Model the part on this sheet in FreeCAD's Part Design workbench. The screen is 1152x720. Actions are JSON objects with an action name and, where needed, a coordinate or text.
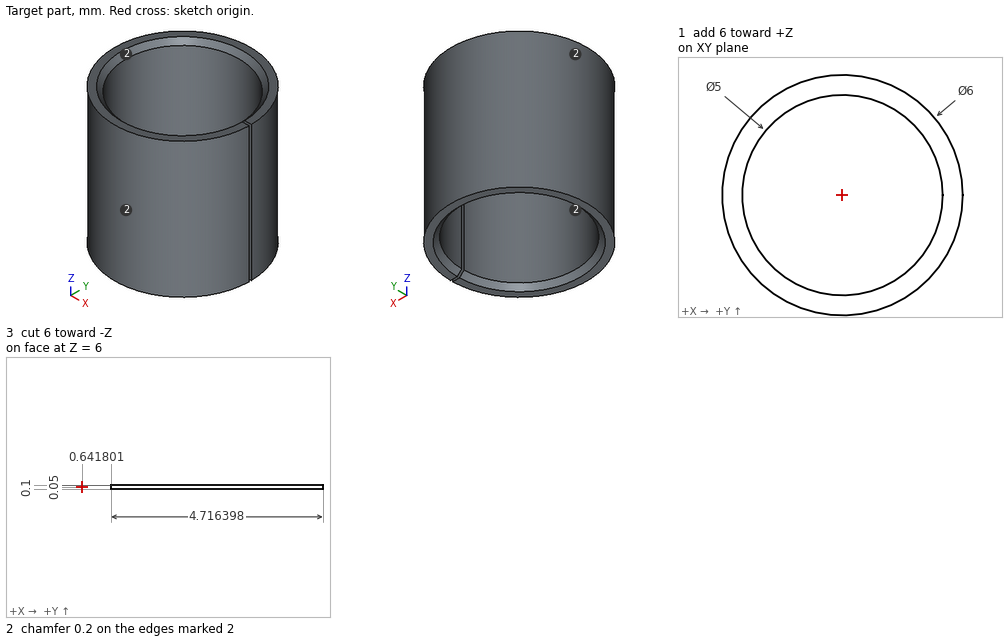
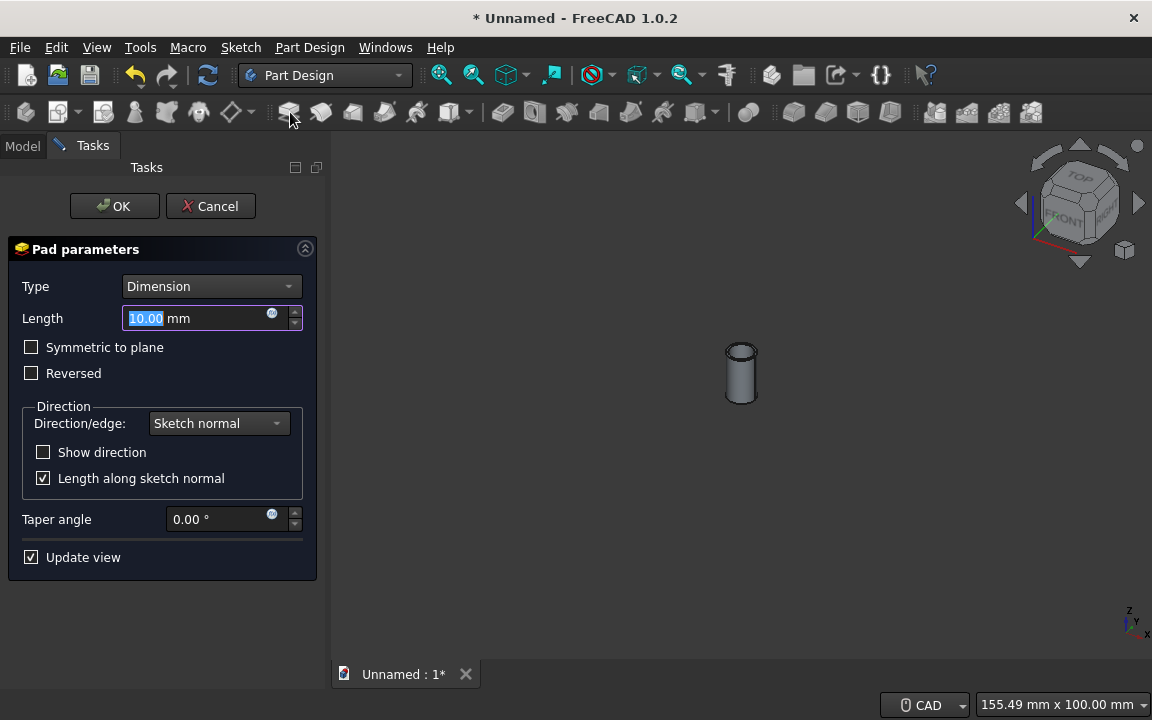
{"action": "type", "text": "6"}
{"action": "key", "text": "Tab"}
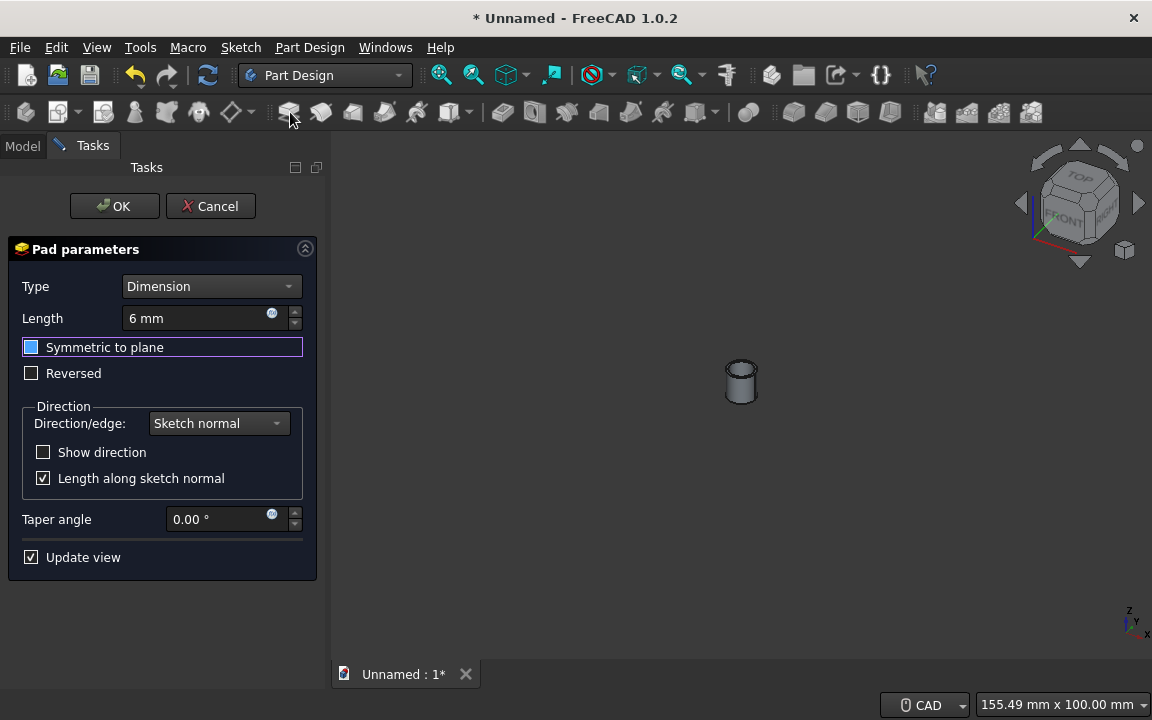
{"action": "left_click", "coordinate": [115, 206]}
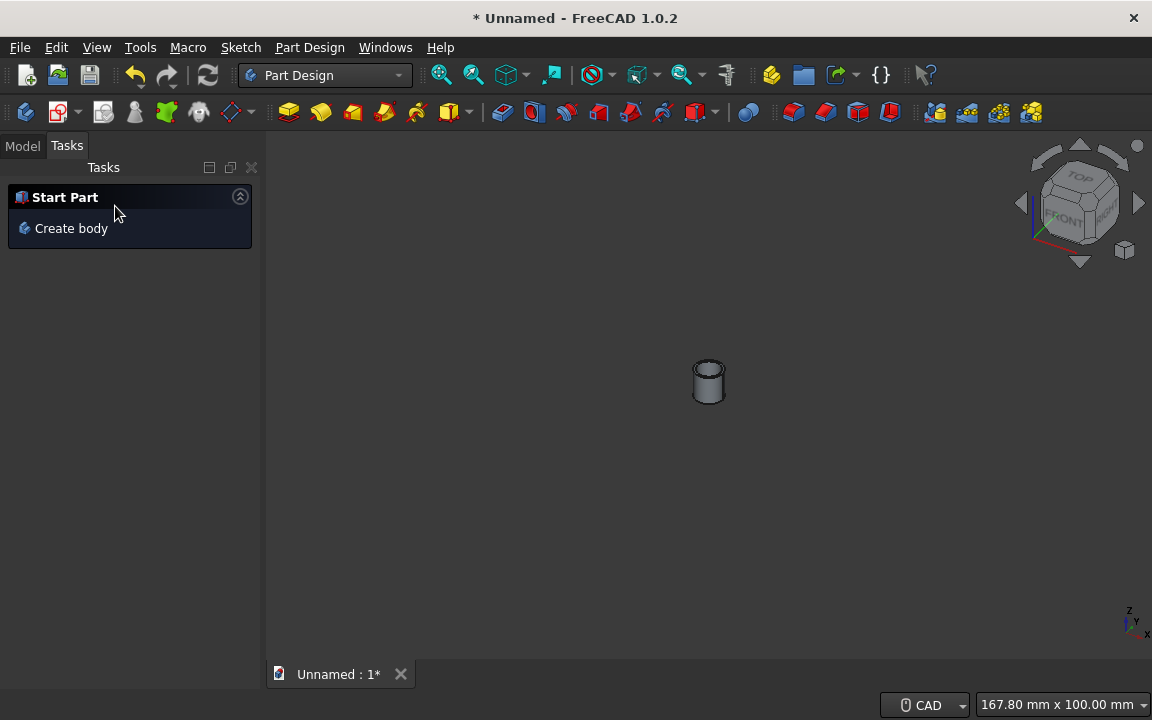
{"action": "left_click", "coordinate": [442, 76]}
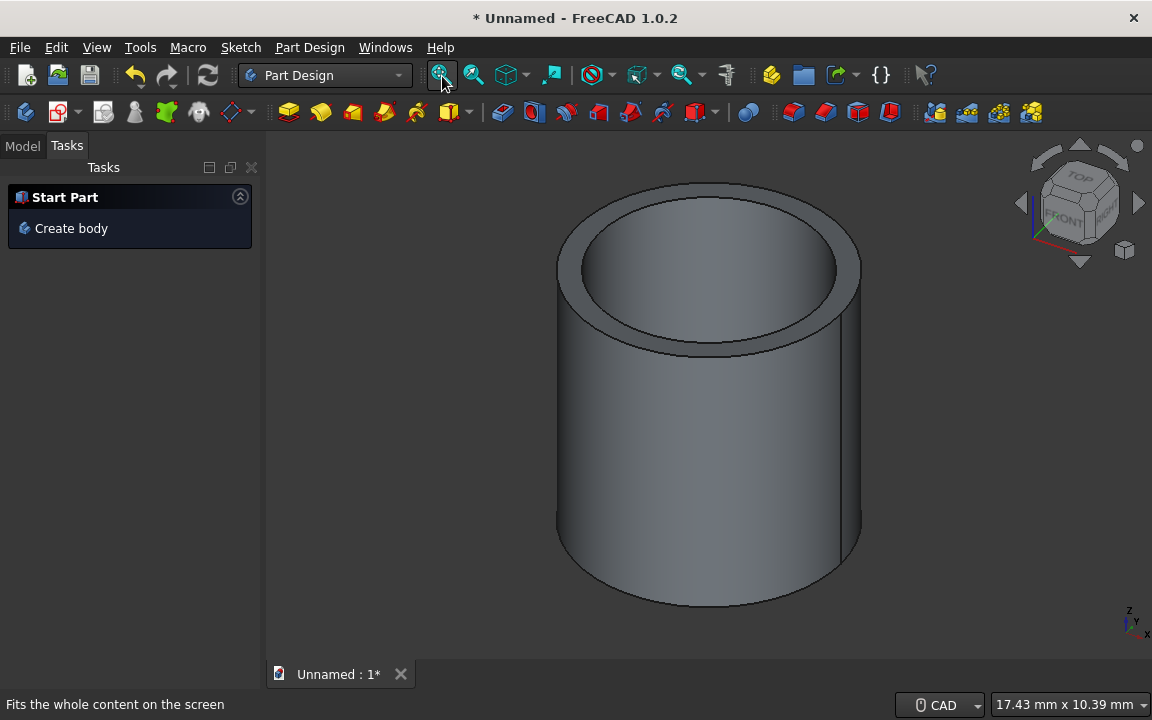
{"action": "left_click", "coordinate": [599, 233]}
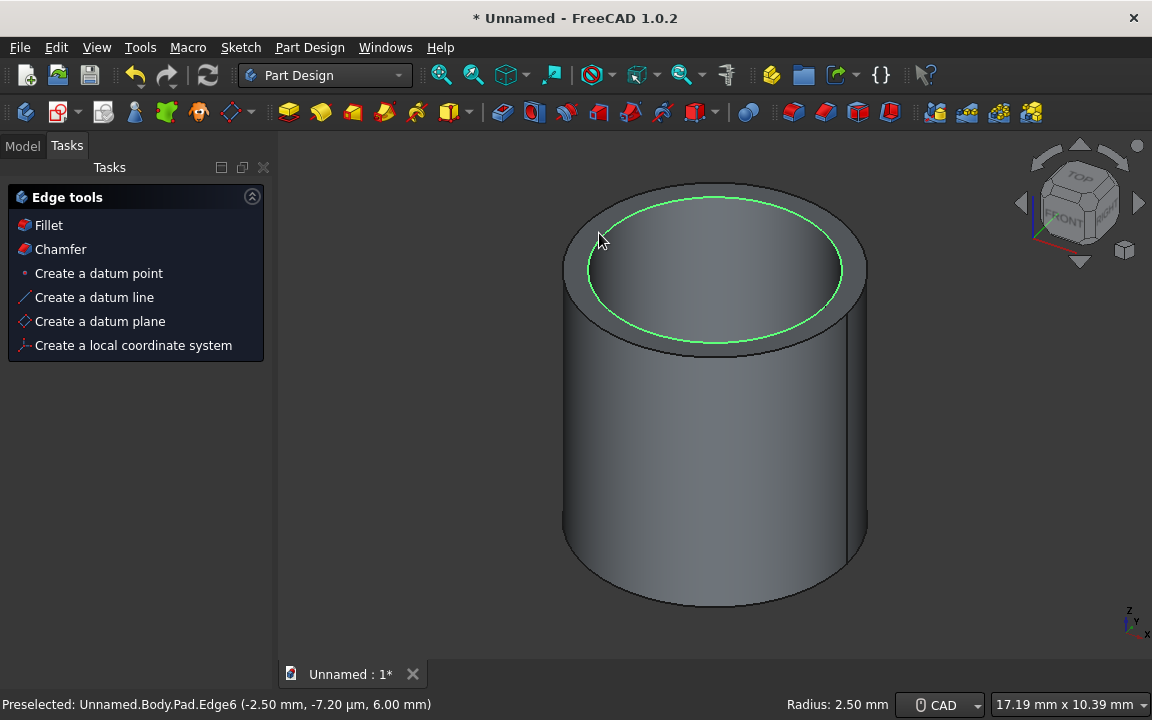
{"action": "key", "text": "0"}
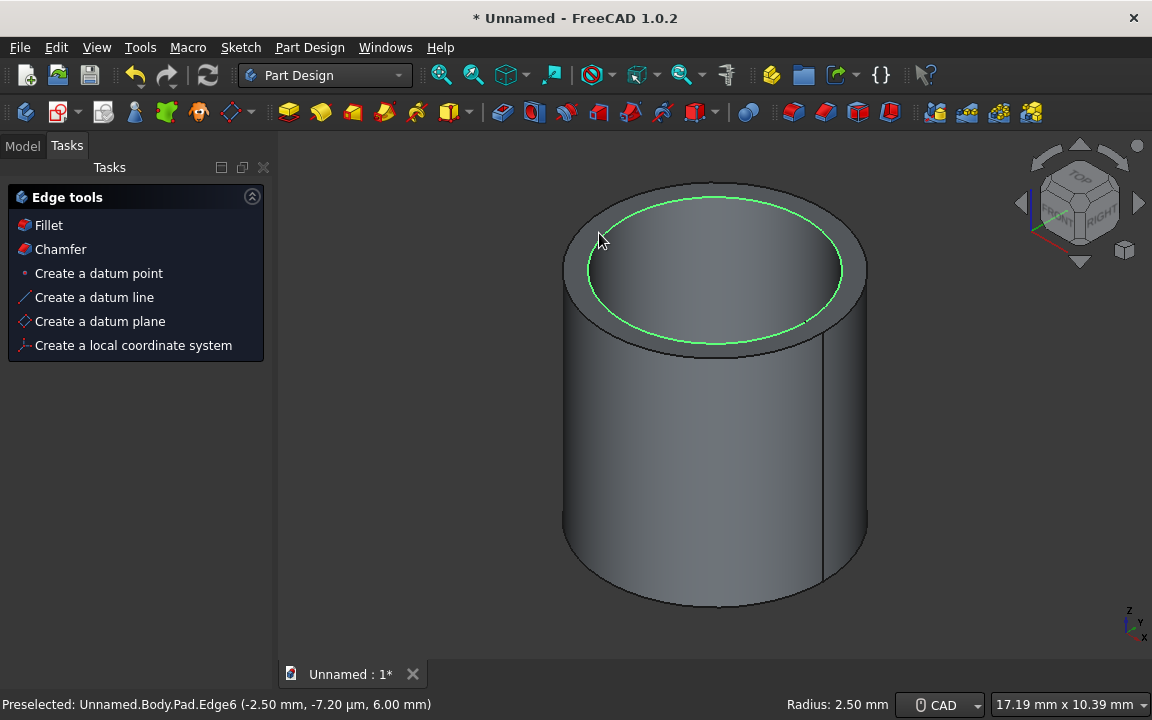
{"action": "key", "text": "2"}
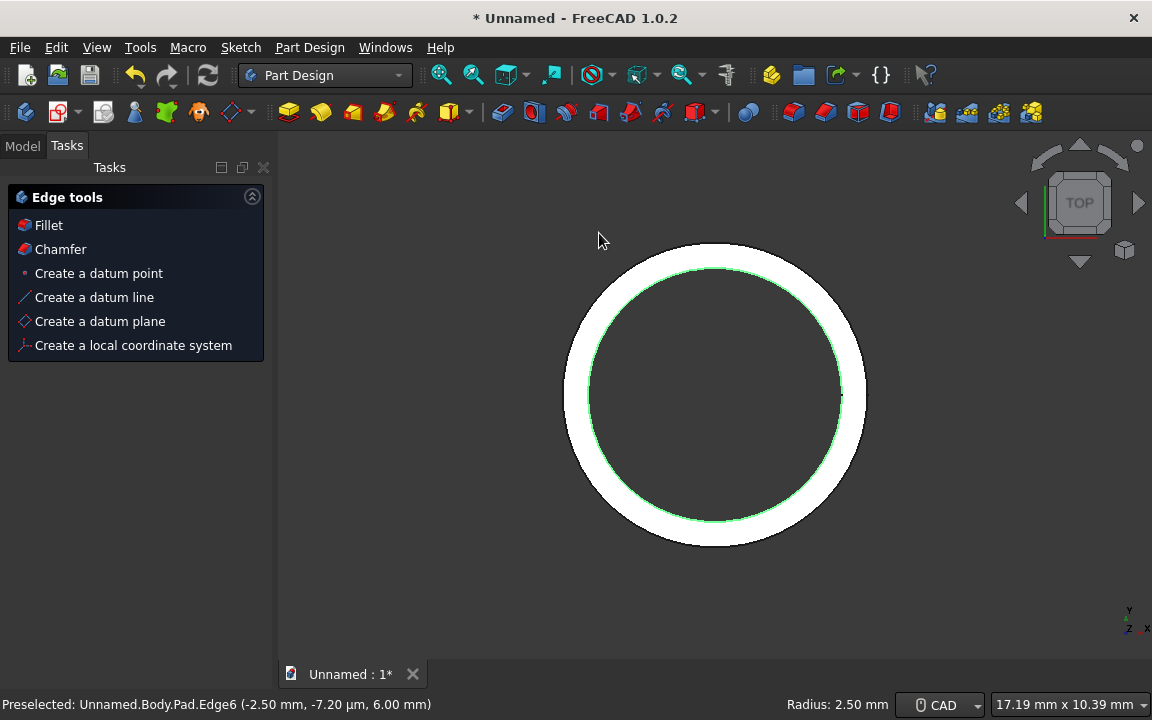
{"action": "key", "text": "1"}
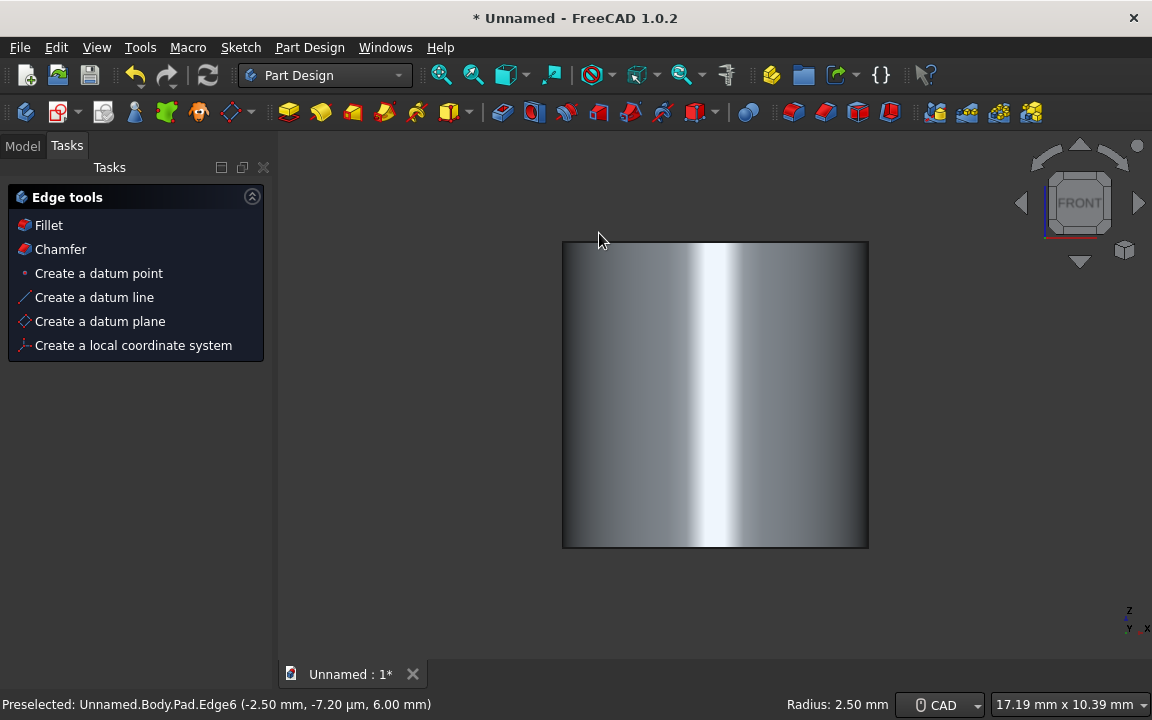
{"action": "key", "text": "3"}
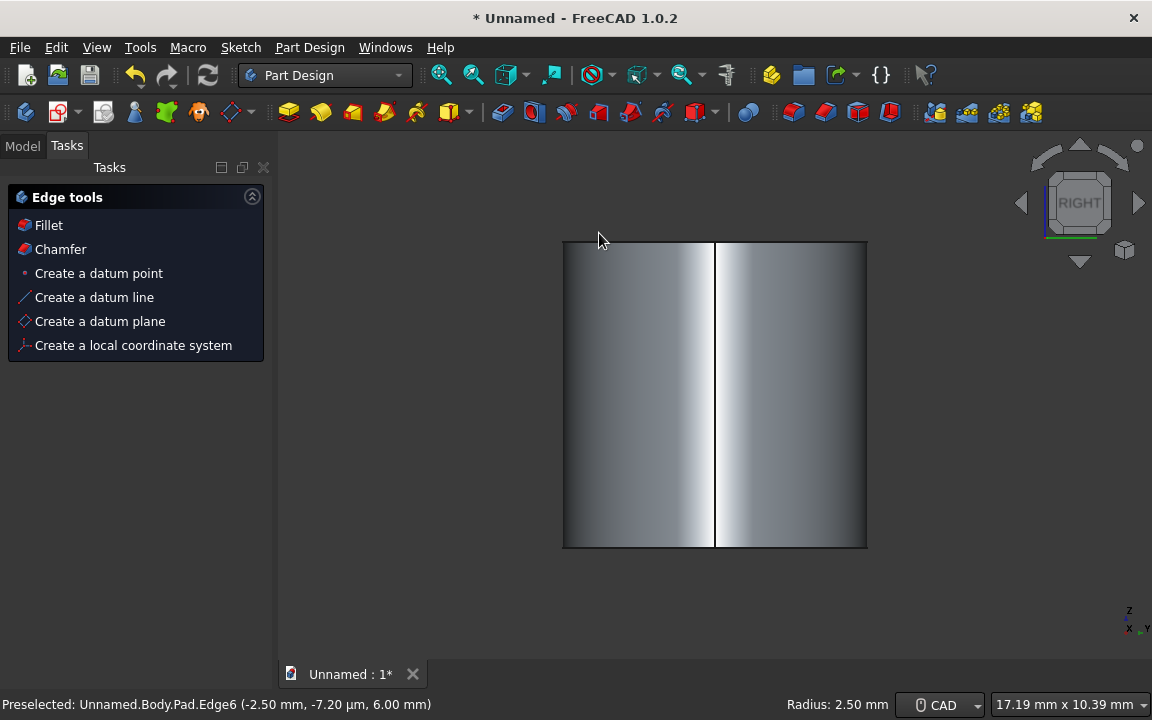
{"action": "key", "text": "5"}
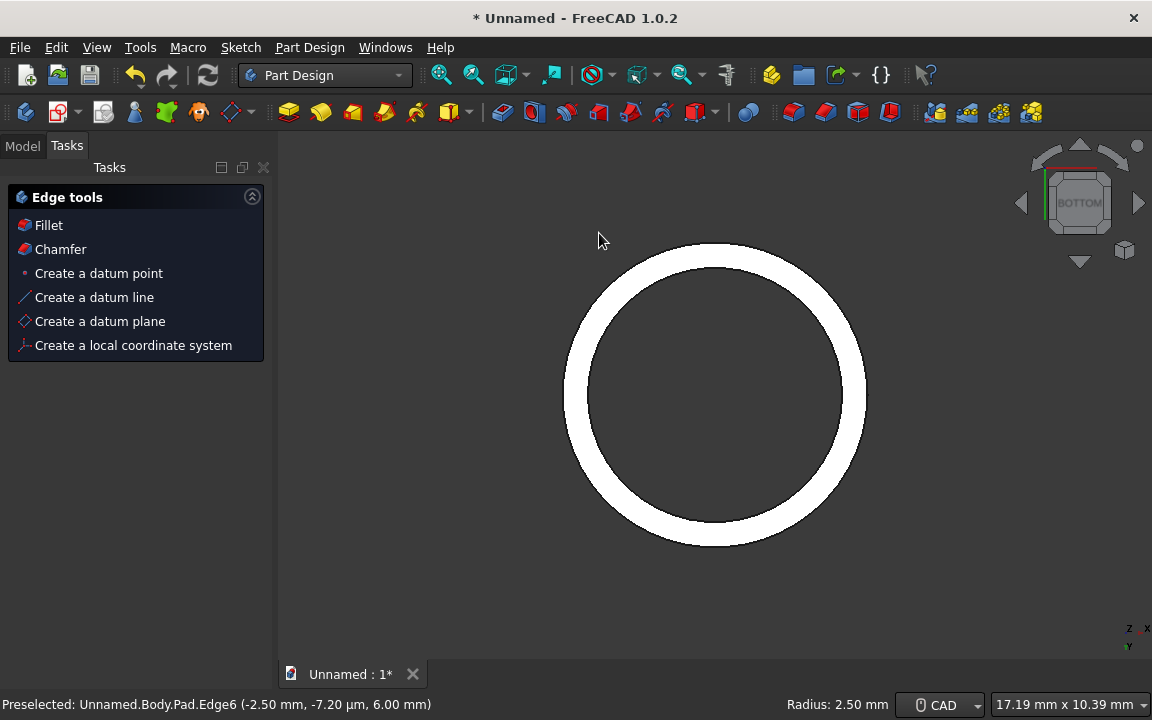
{"action": "left_click", "coordinate": [588, 394], "text": "ctrl"}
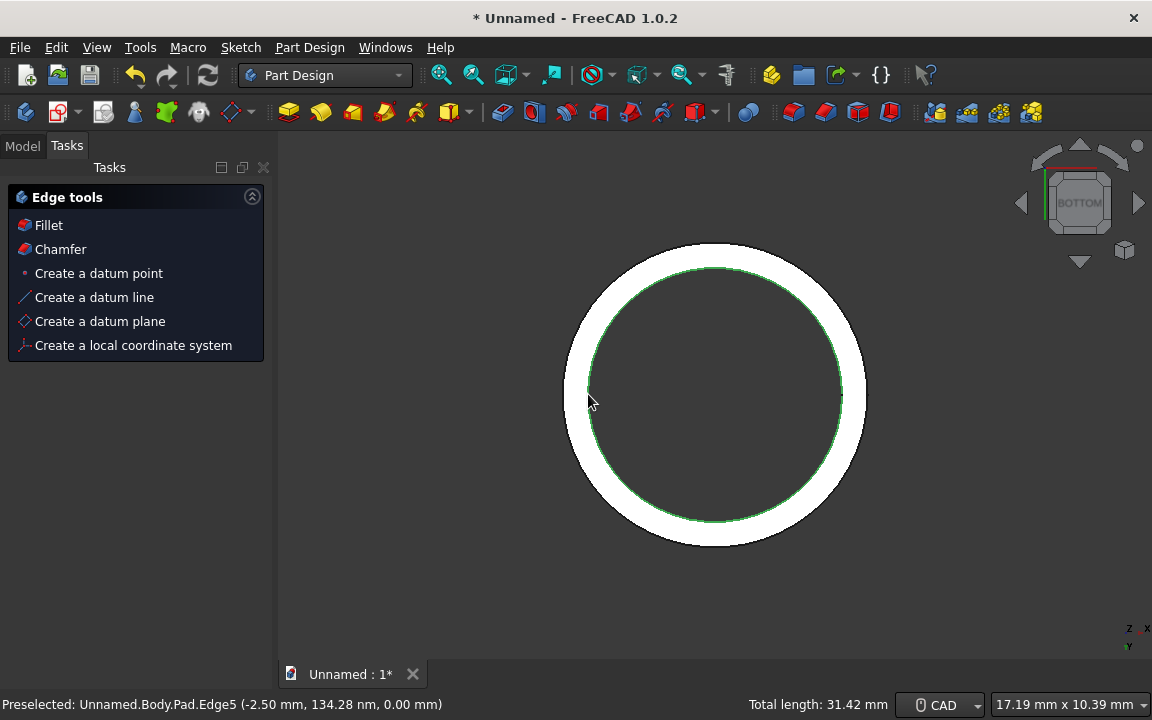
{"action": "left_click", "coordinate": [826, 112]}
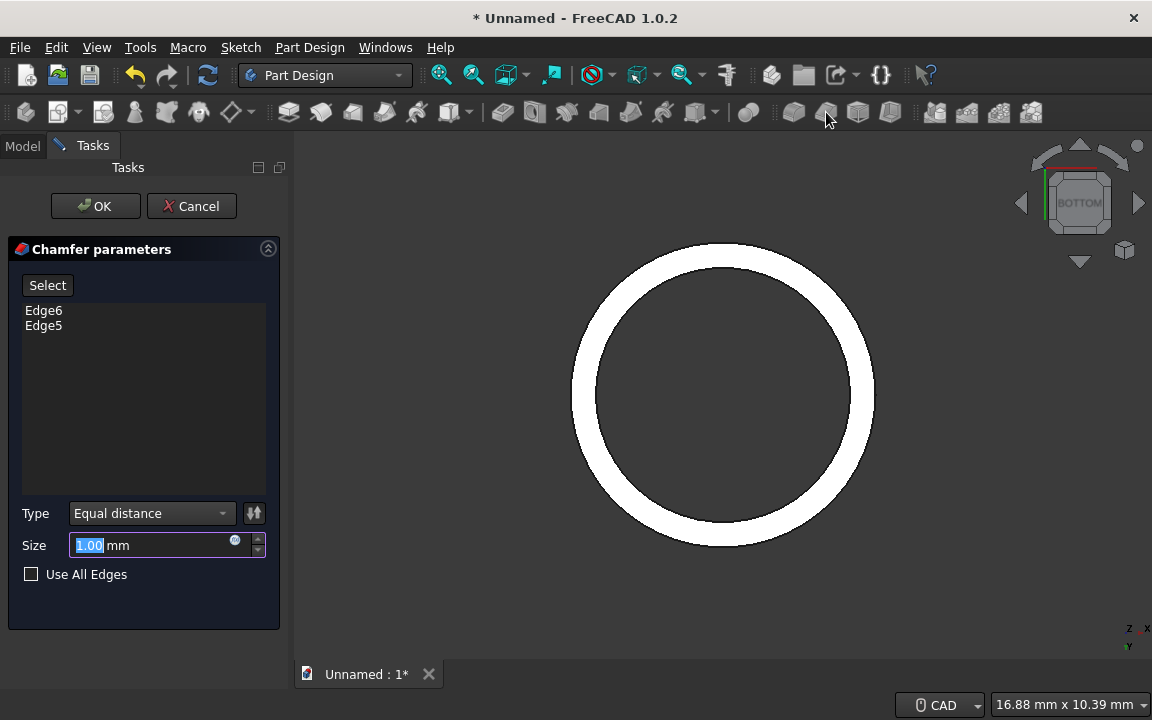
{"action": "type", "text": "0.2"}
{"action": "key", "text": "Tab"}